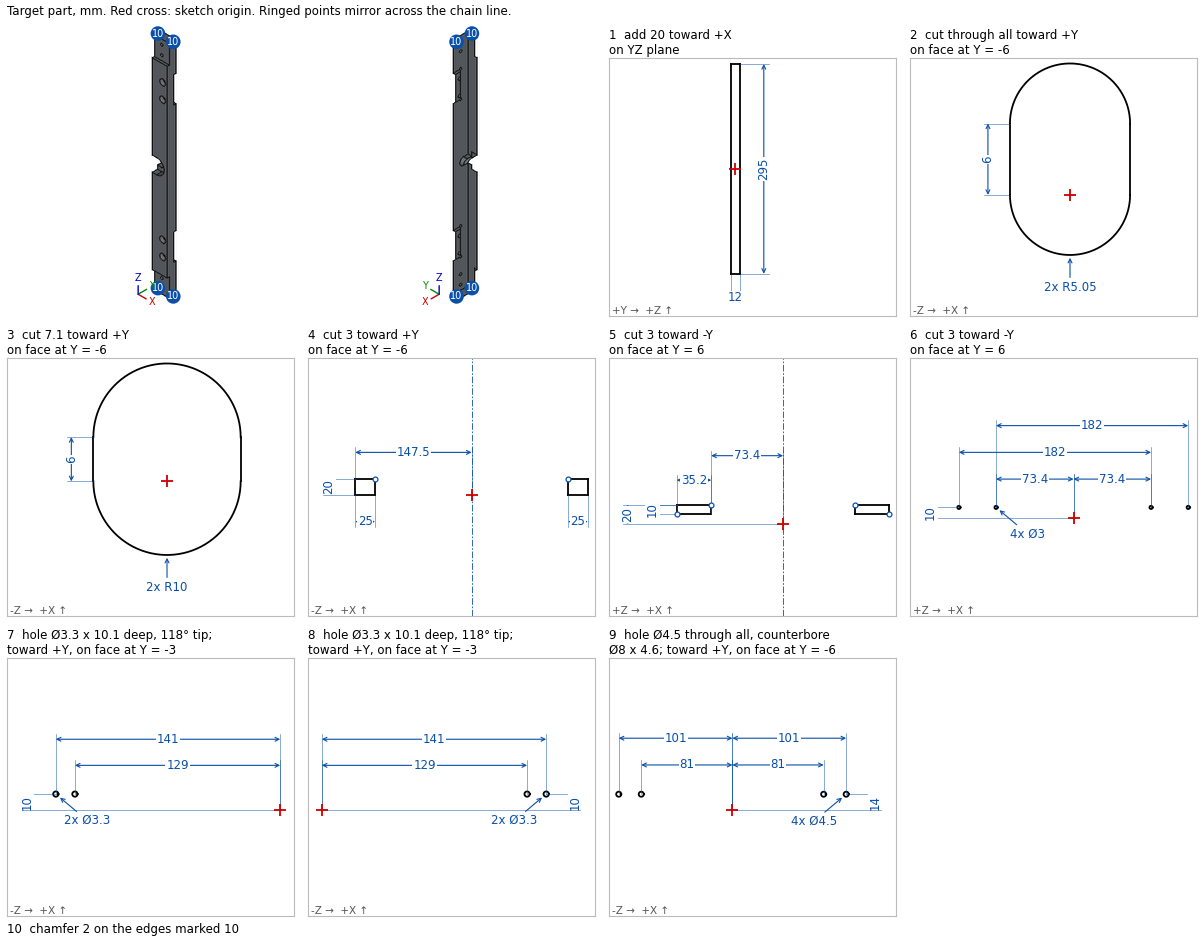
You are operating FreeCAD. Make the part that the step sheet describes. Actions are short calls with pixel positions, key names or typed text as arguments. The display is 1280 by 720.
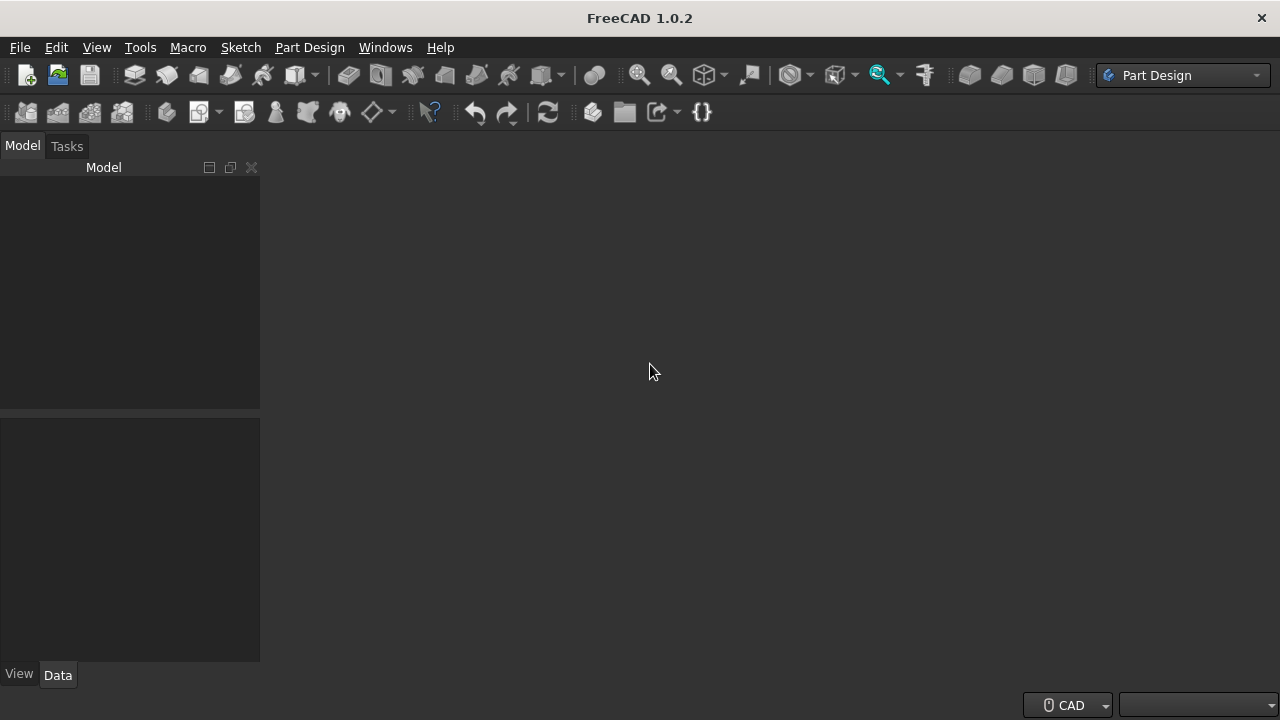
click(26, 76)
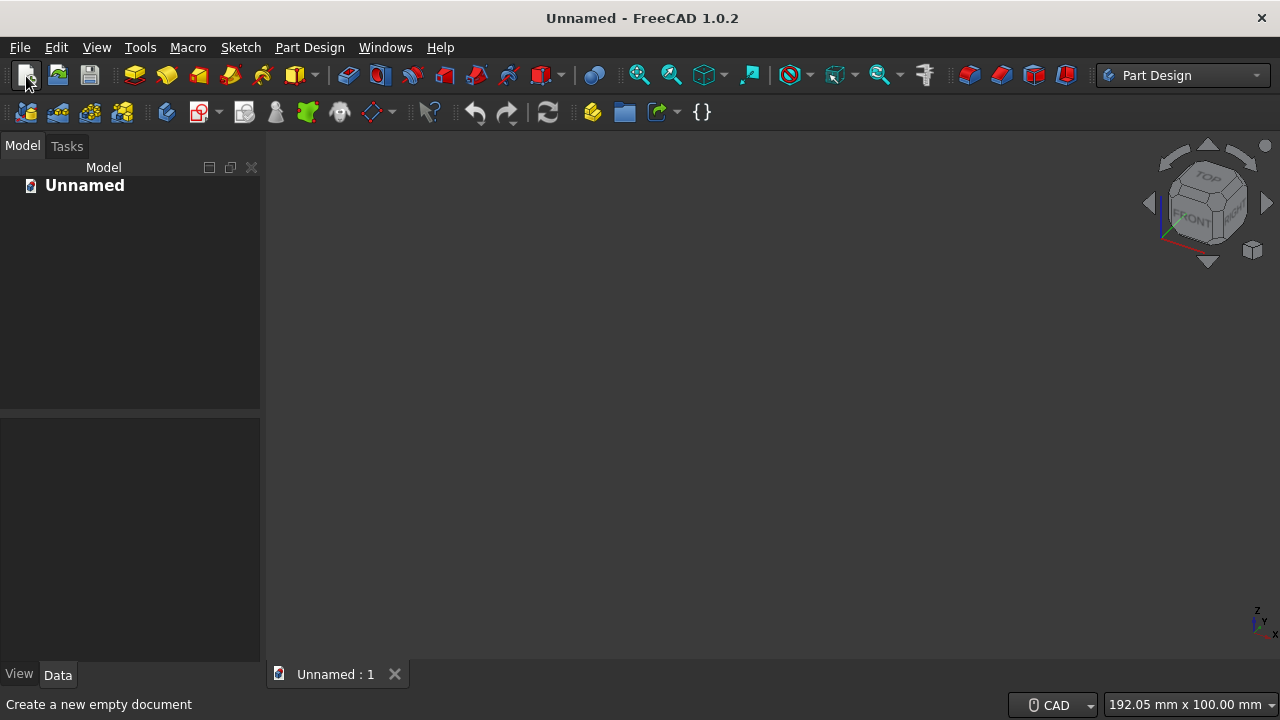
click(200, 112)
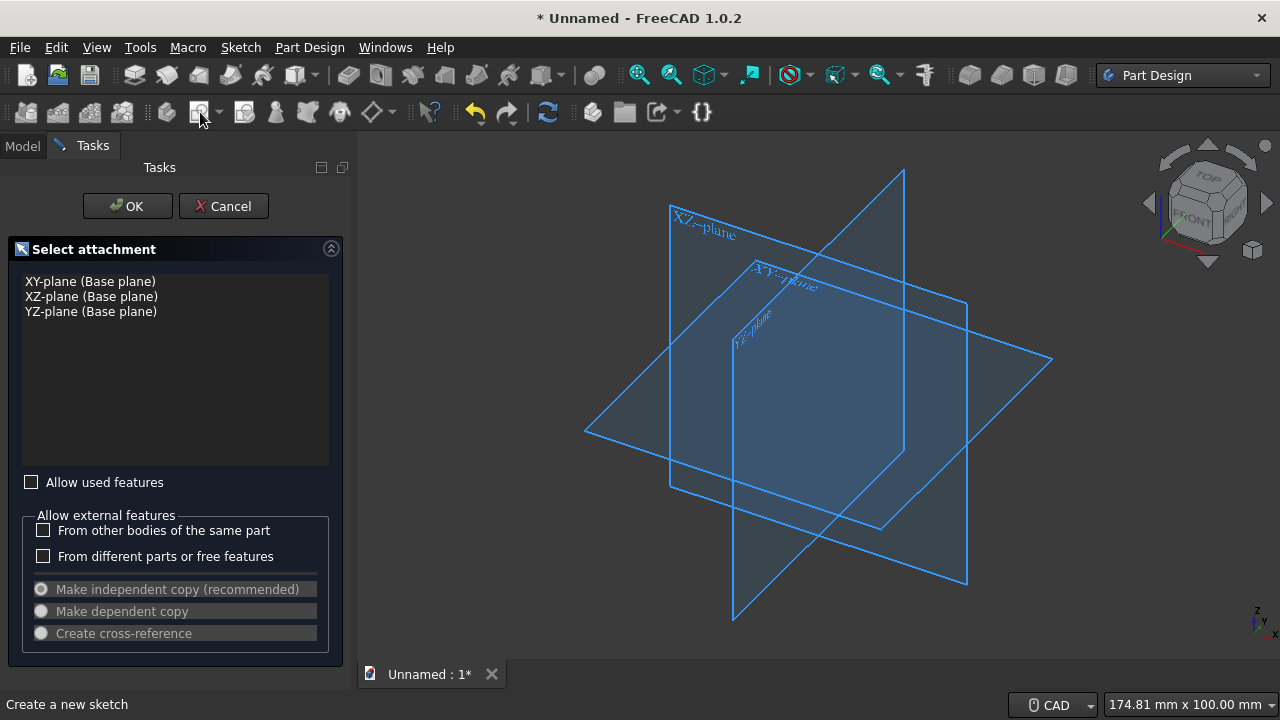
click(82, 312)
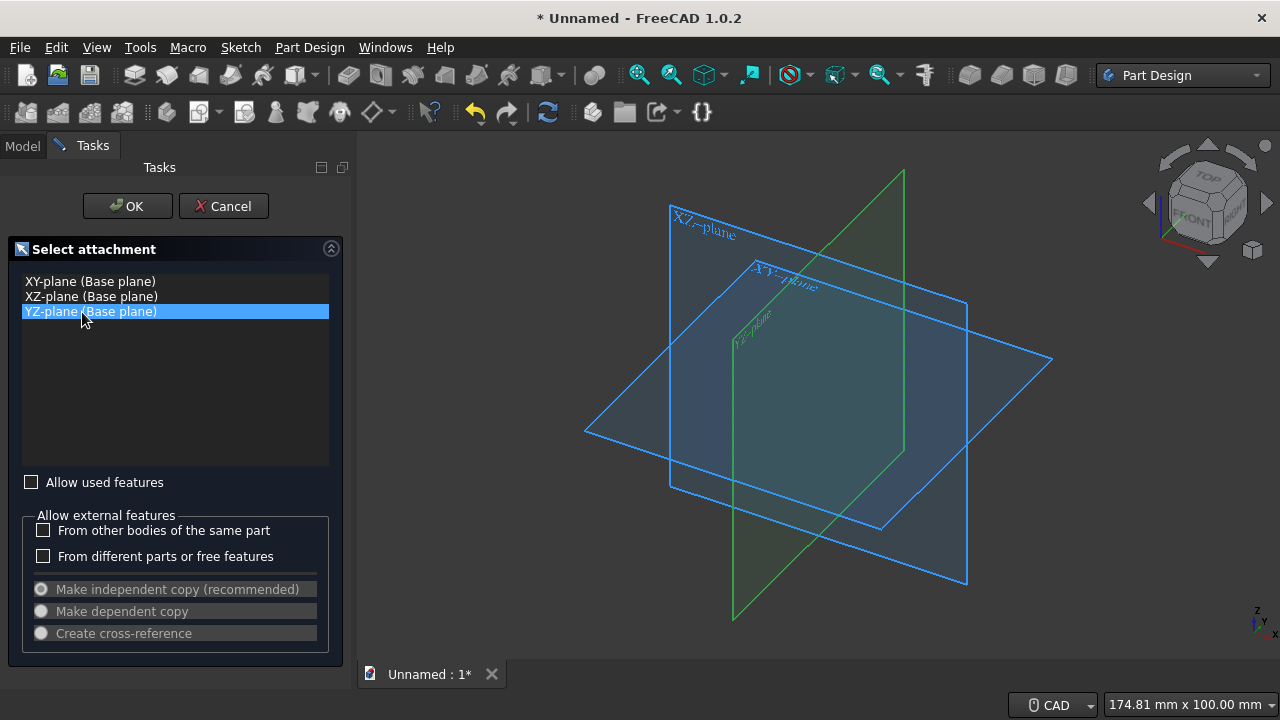
click(128, 206)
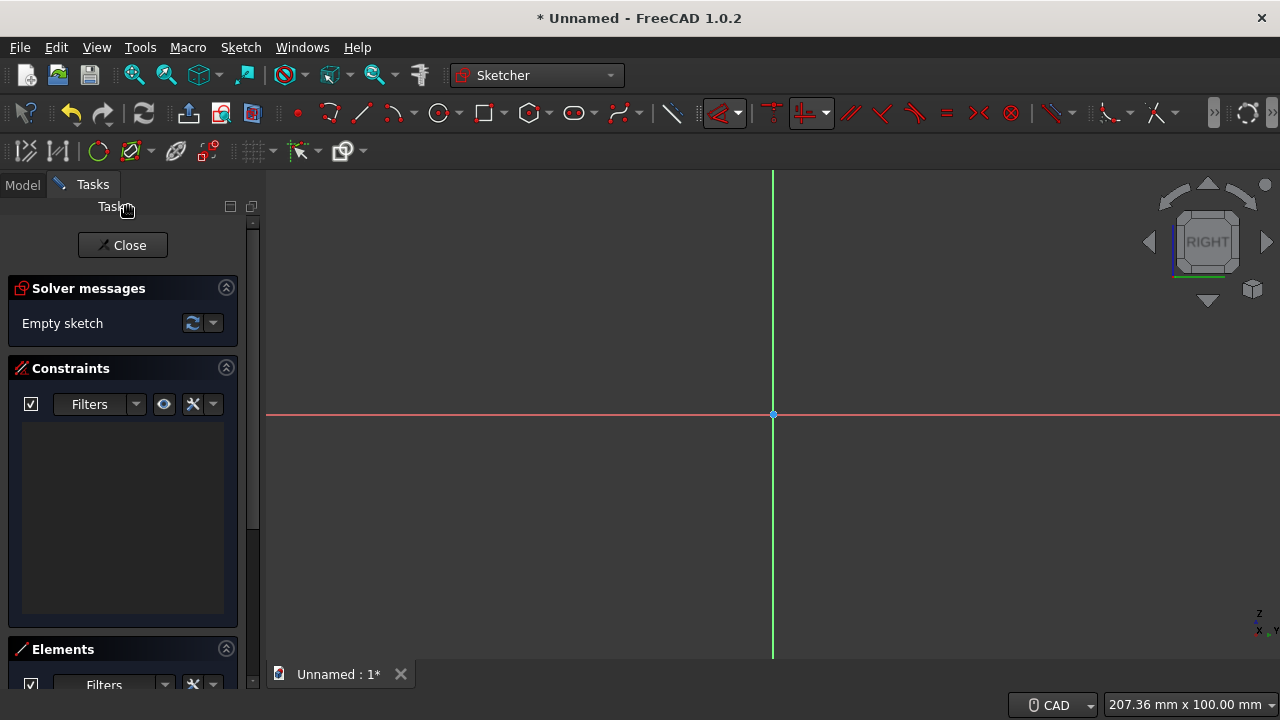
scroll(687, 414, down, 8)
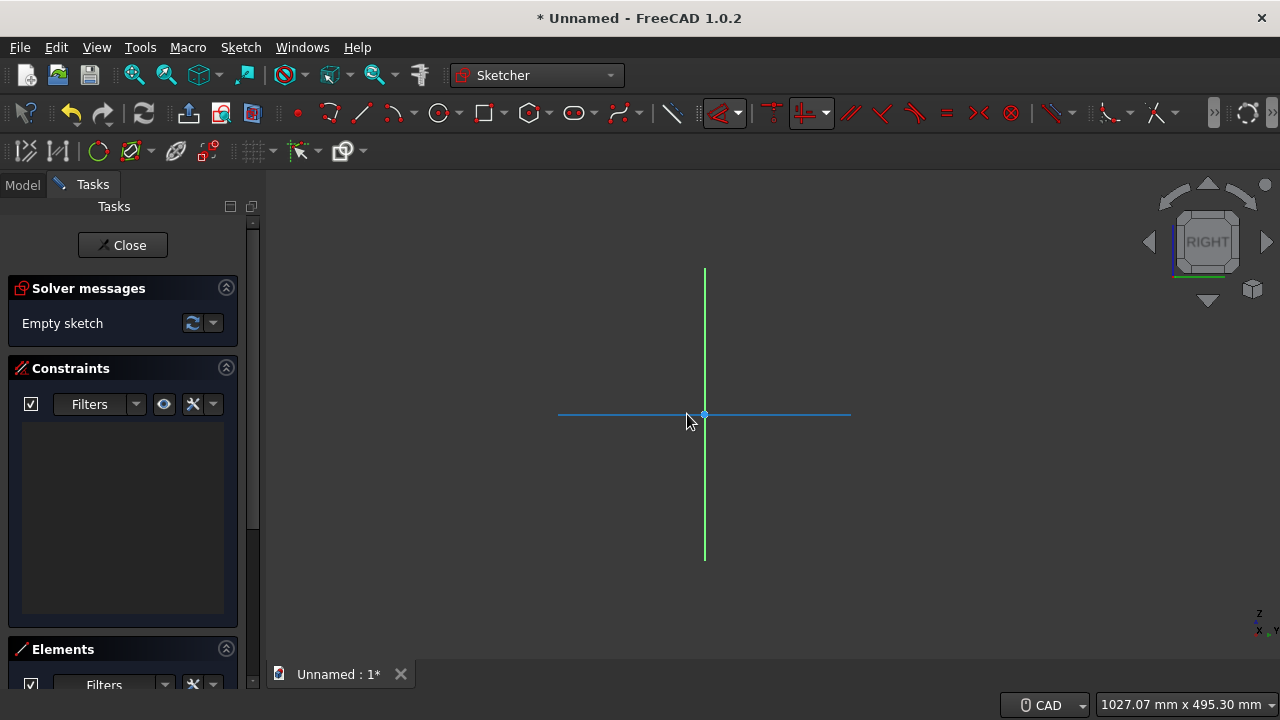
key(g)
key(v)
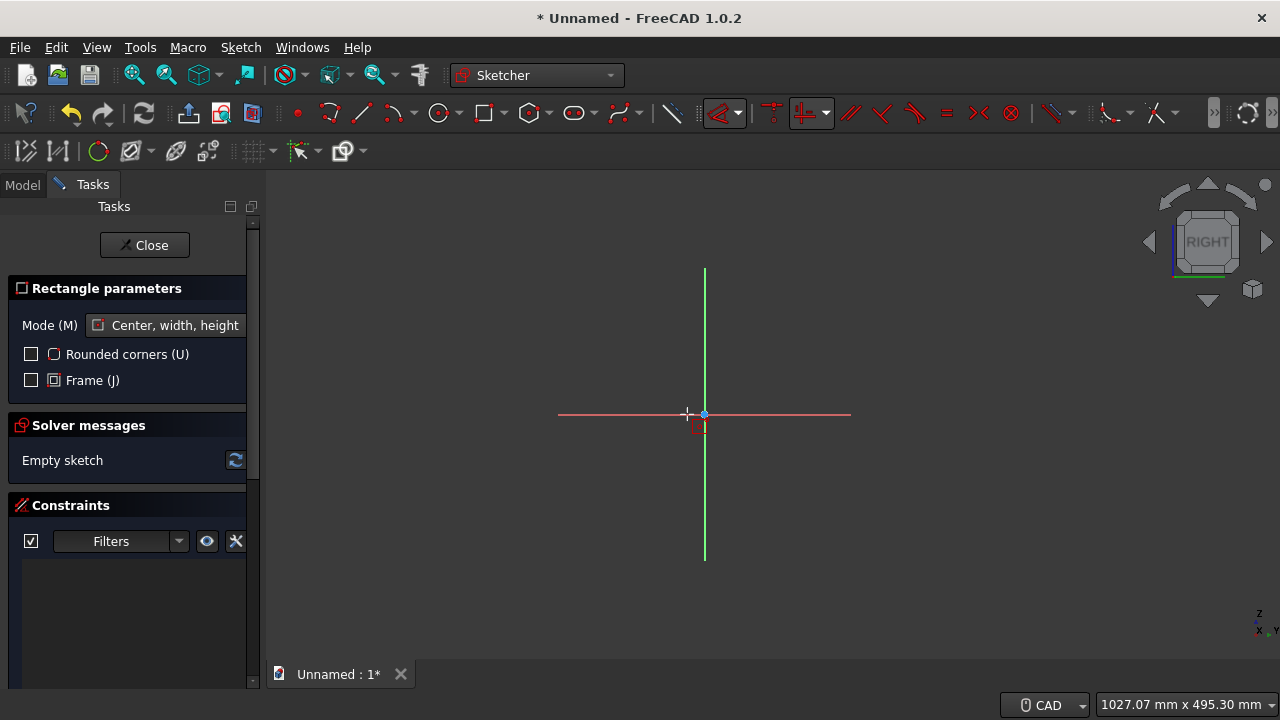
scroll(705, 414, up, 5)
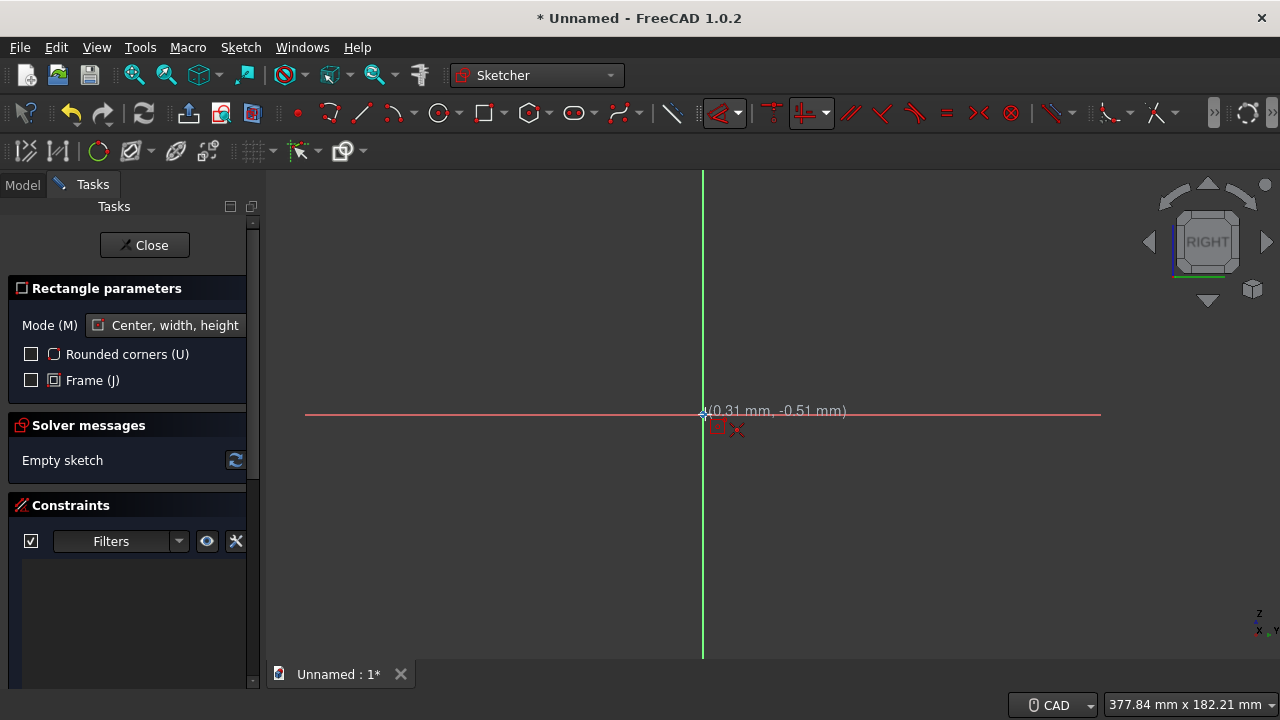
click(703, 414)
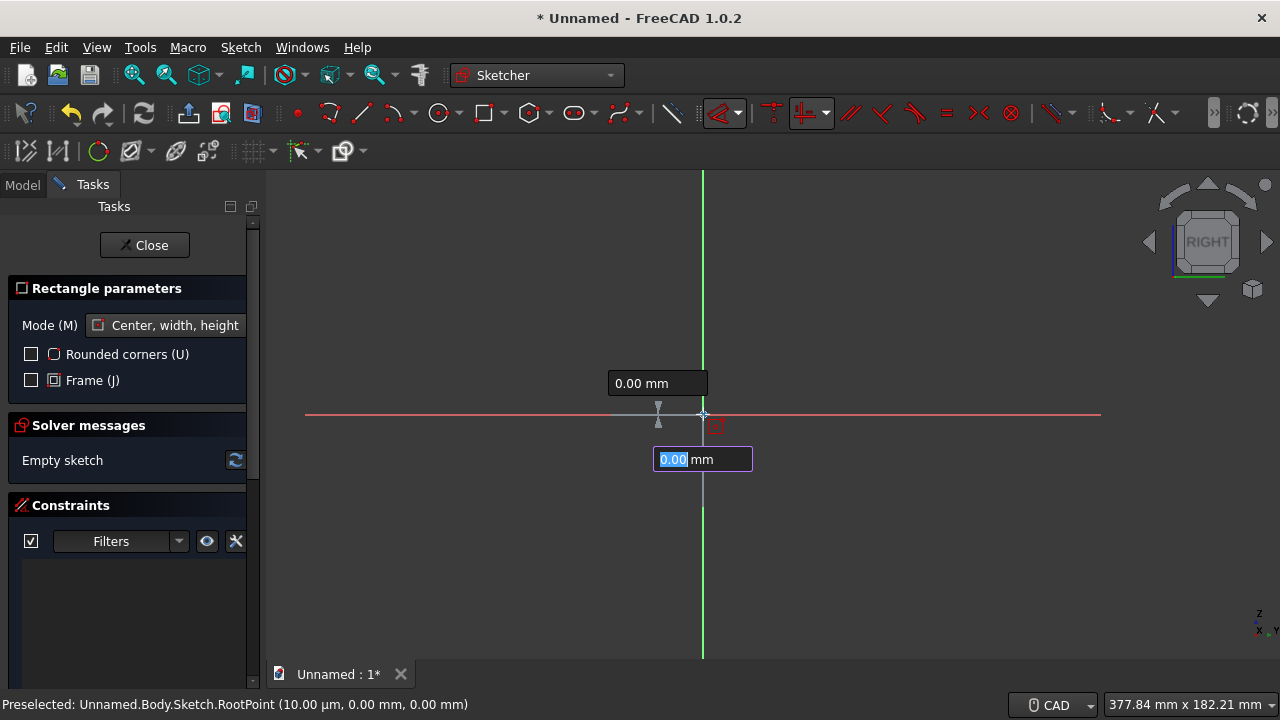
scroll(705, 414, down, 5)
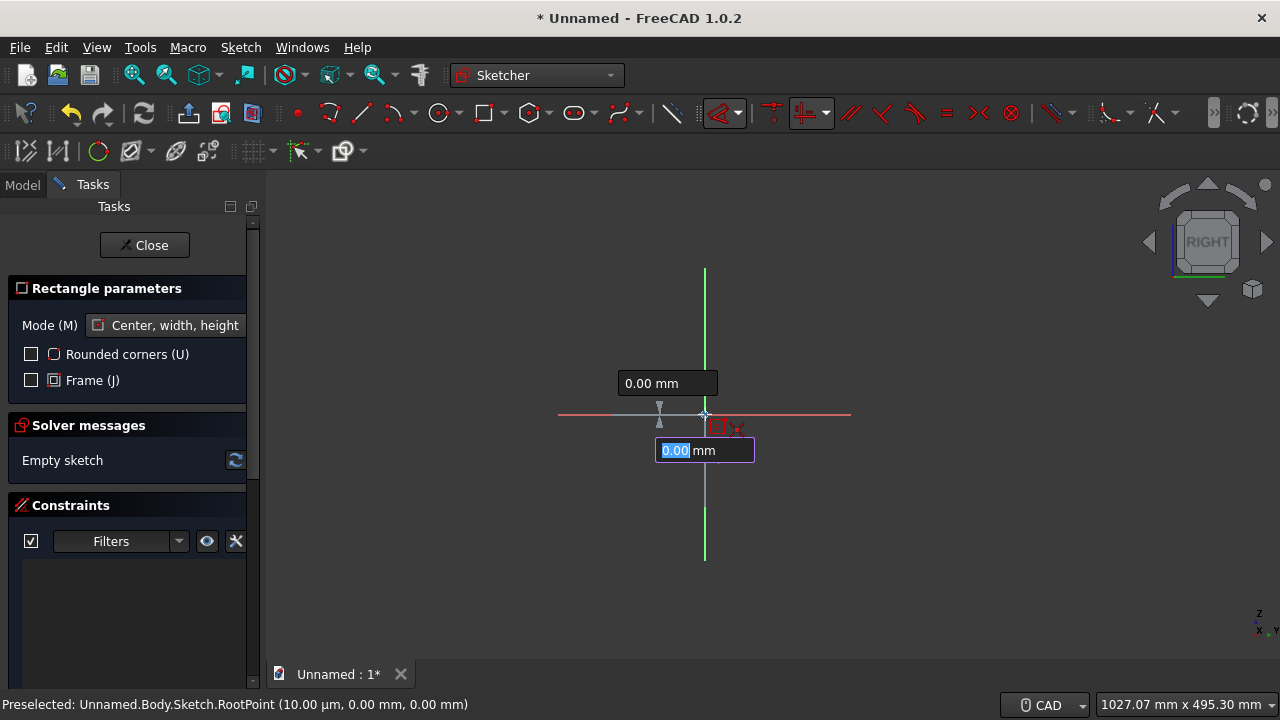
scroll(711, 269, up, 5)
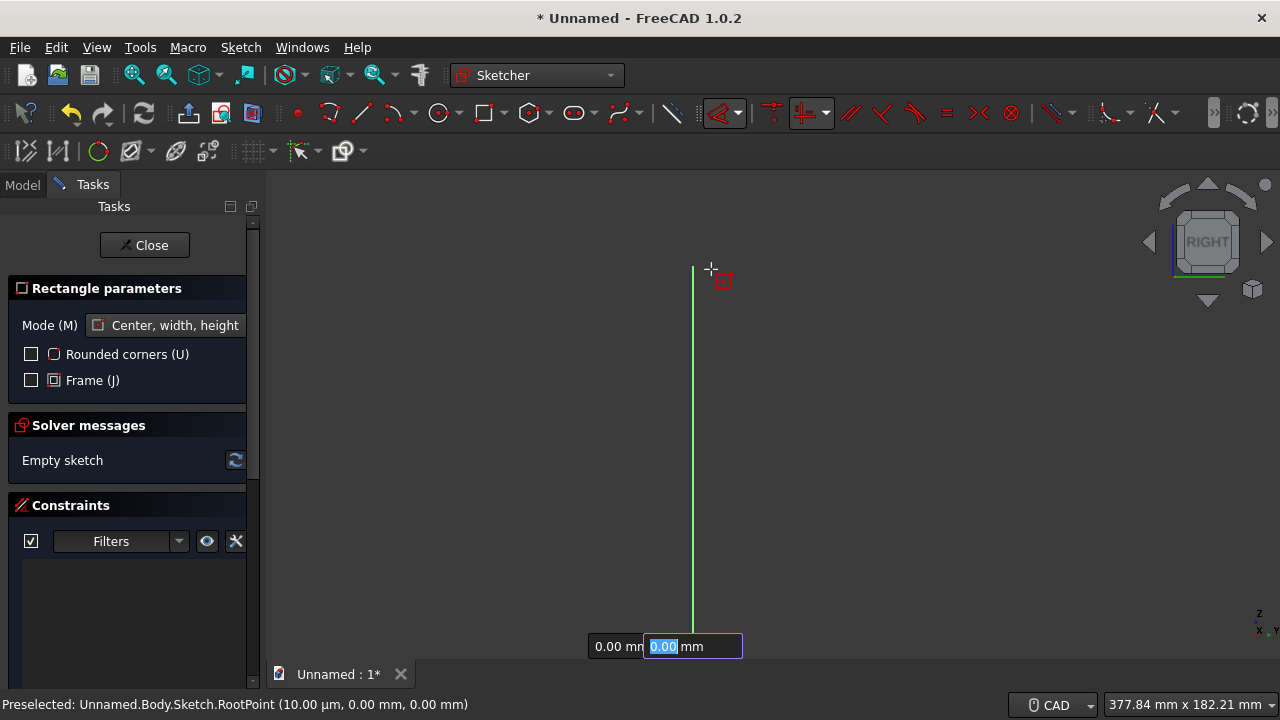
click(709, 268)
key(Escape)